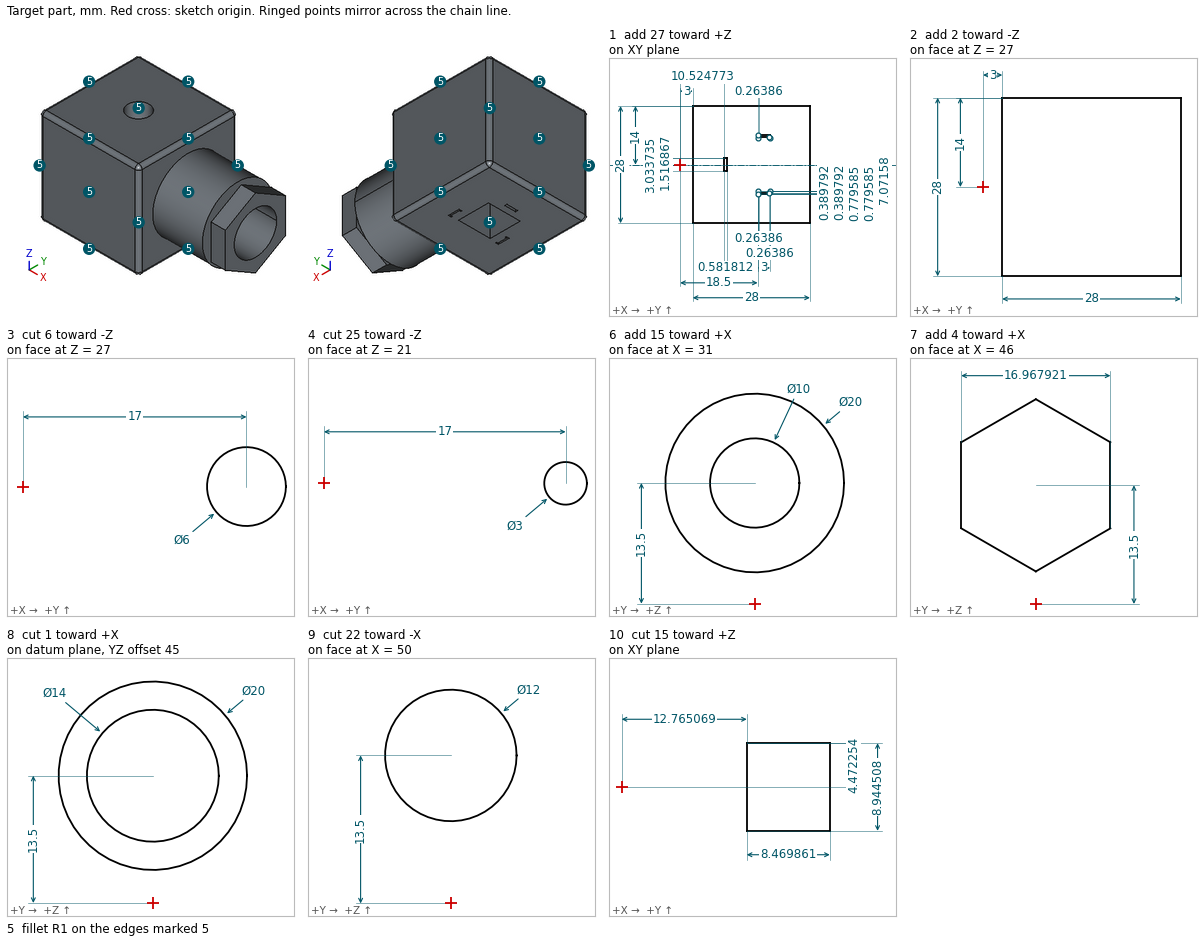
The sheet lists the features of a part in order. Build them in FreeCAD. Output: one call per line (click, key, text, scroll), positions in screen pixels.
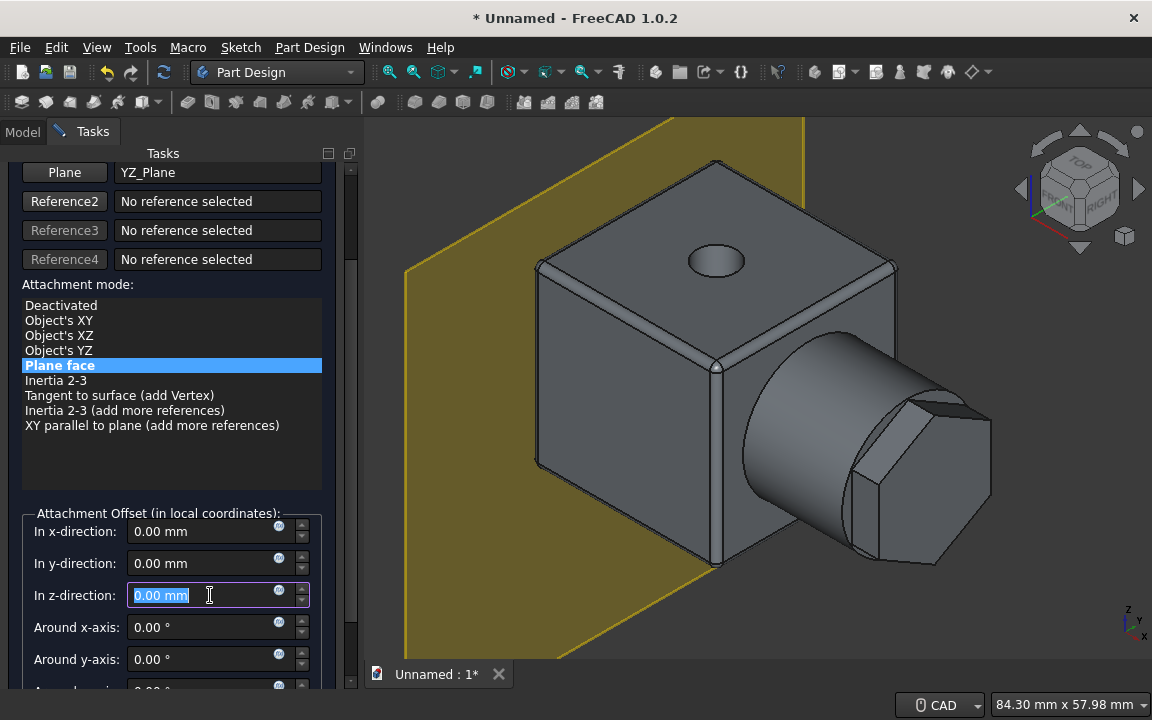
text(45)
key(Tab)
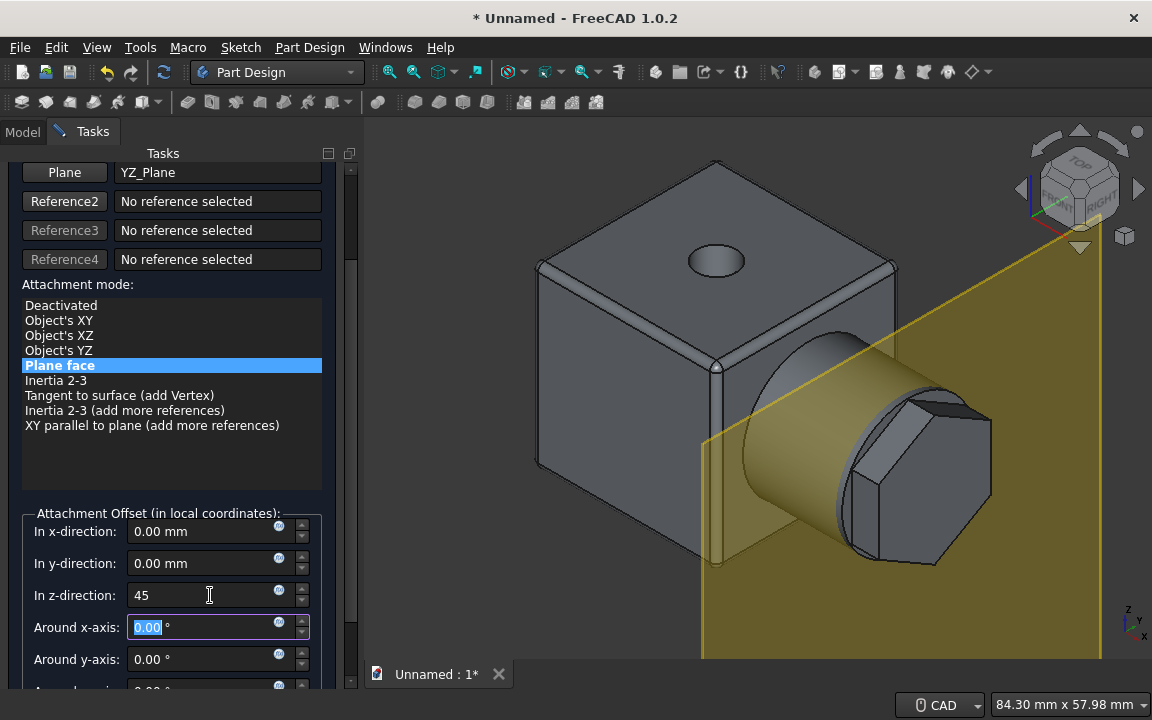
scroll(351, 426, up, 3)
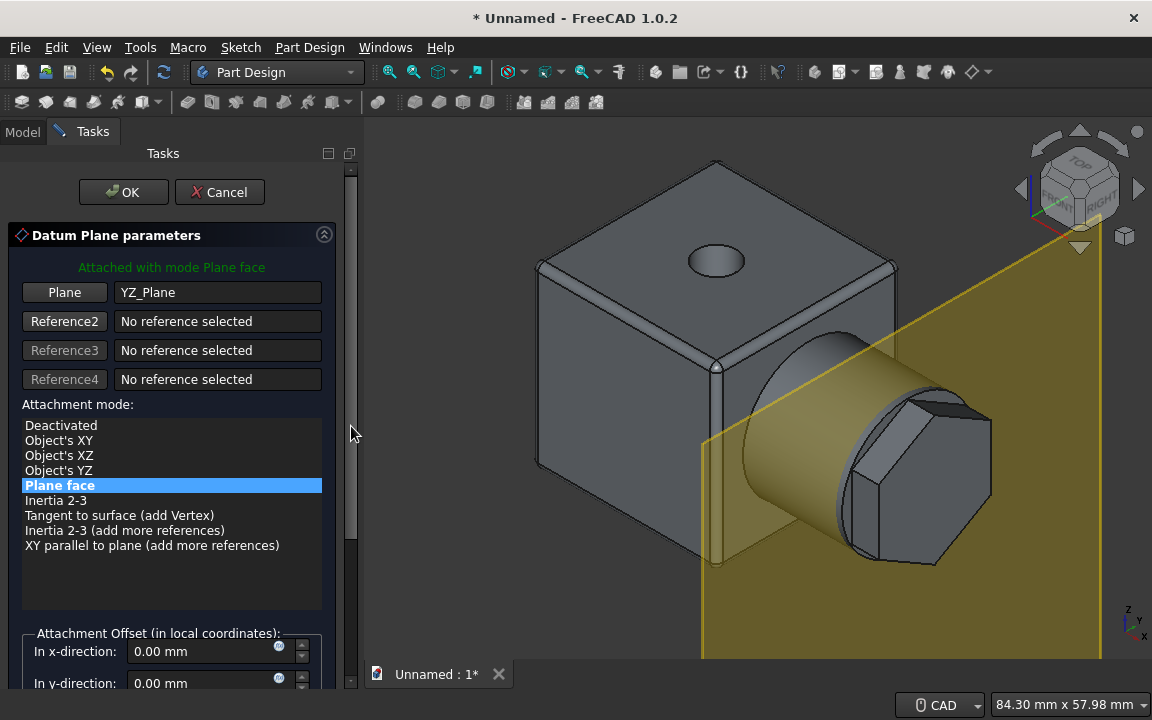
click(124, 192)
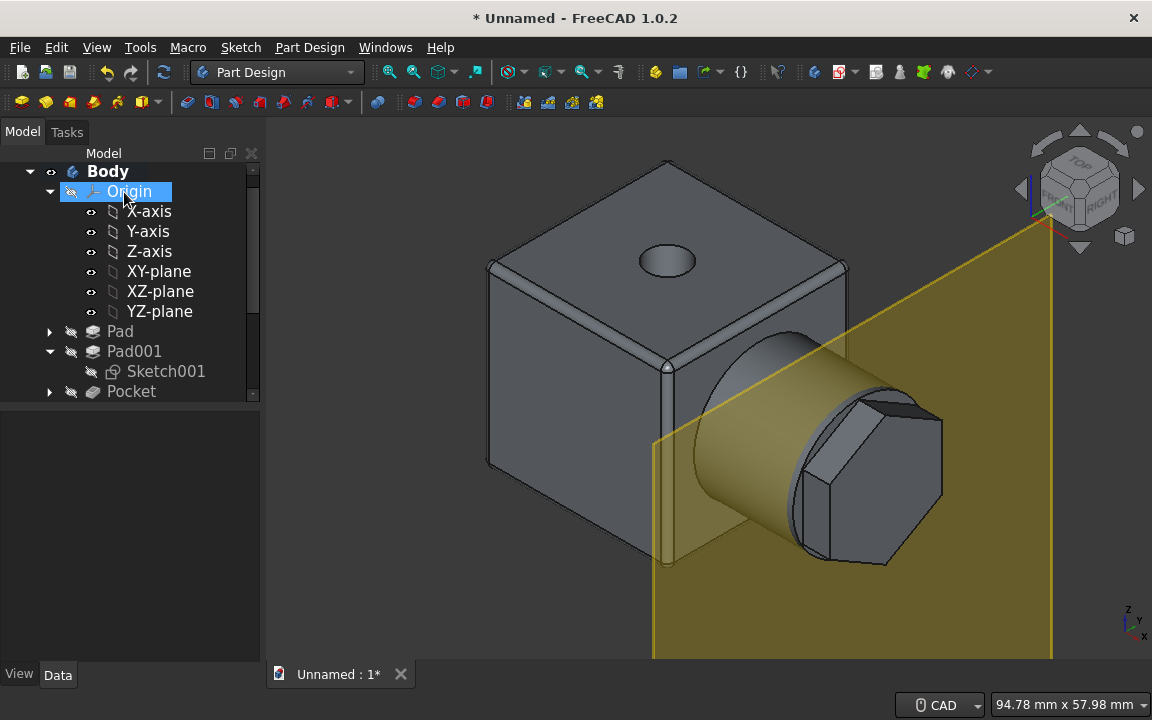
scroll(120, 287, down, 3)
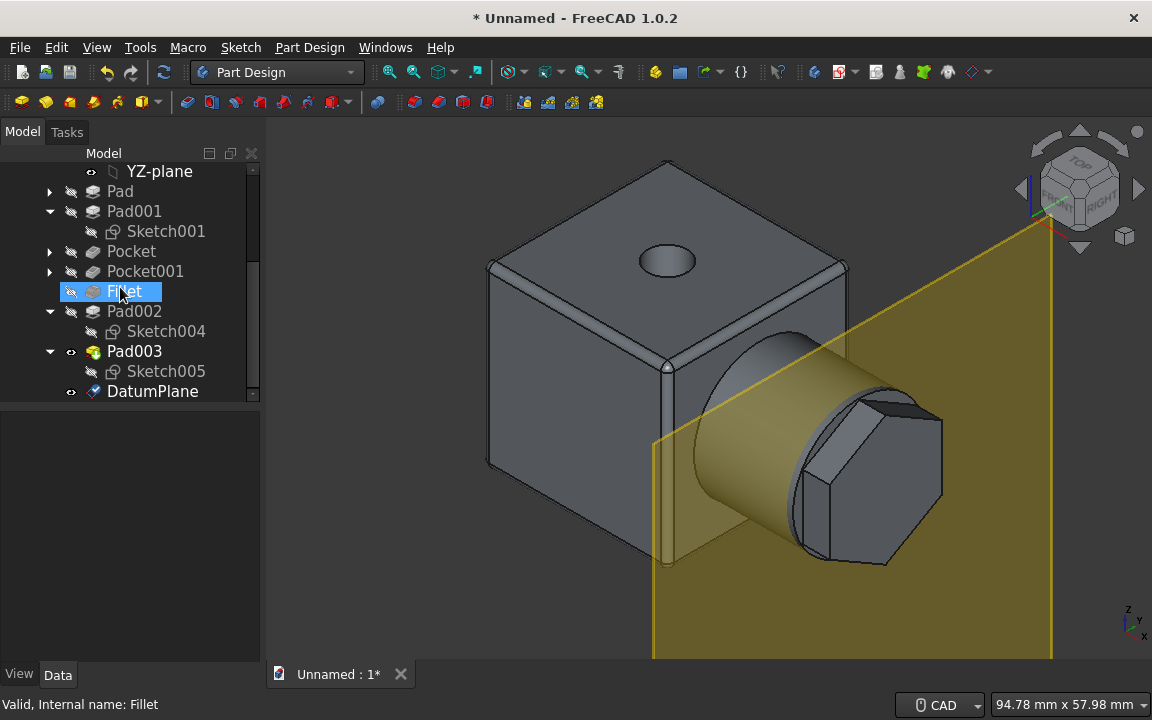
click(116, 392)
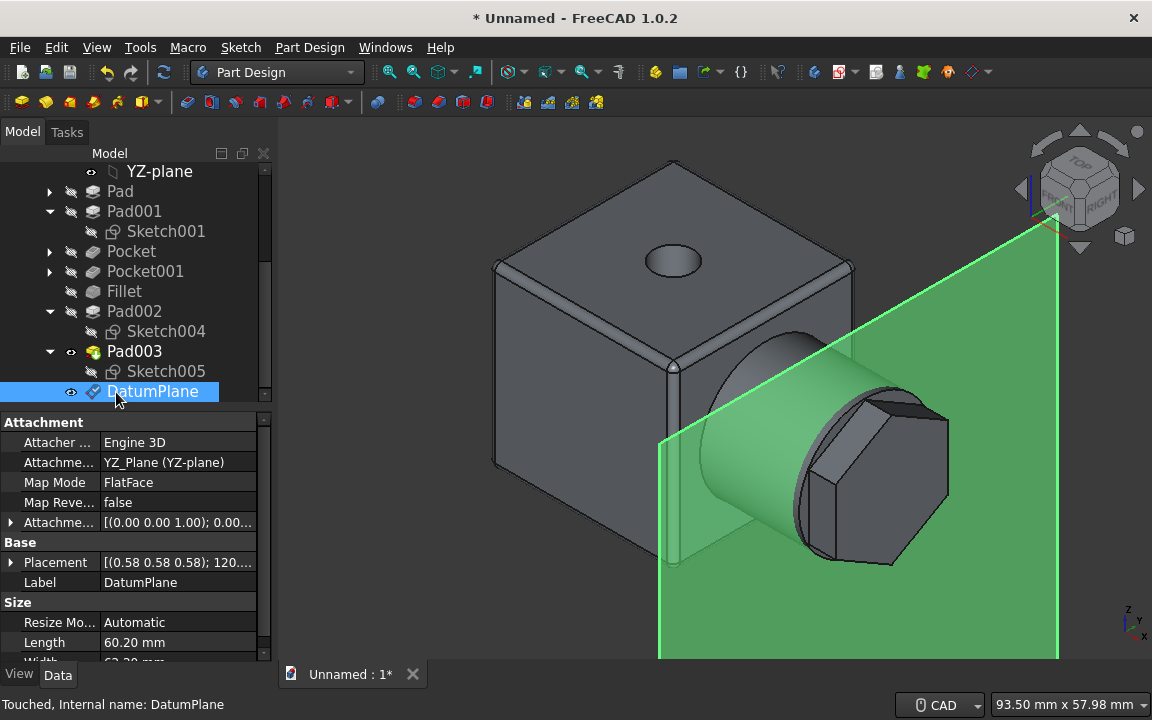
click(840, 72)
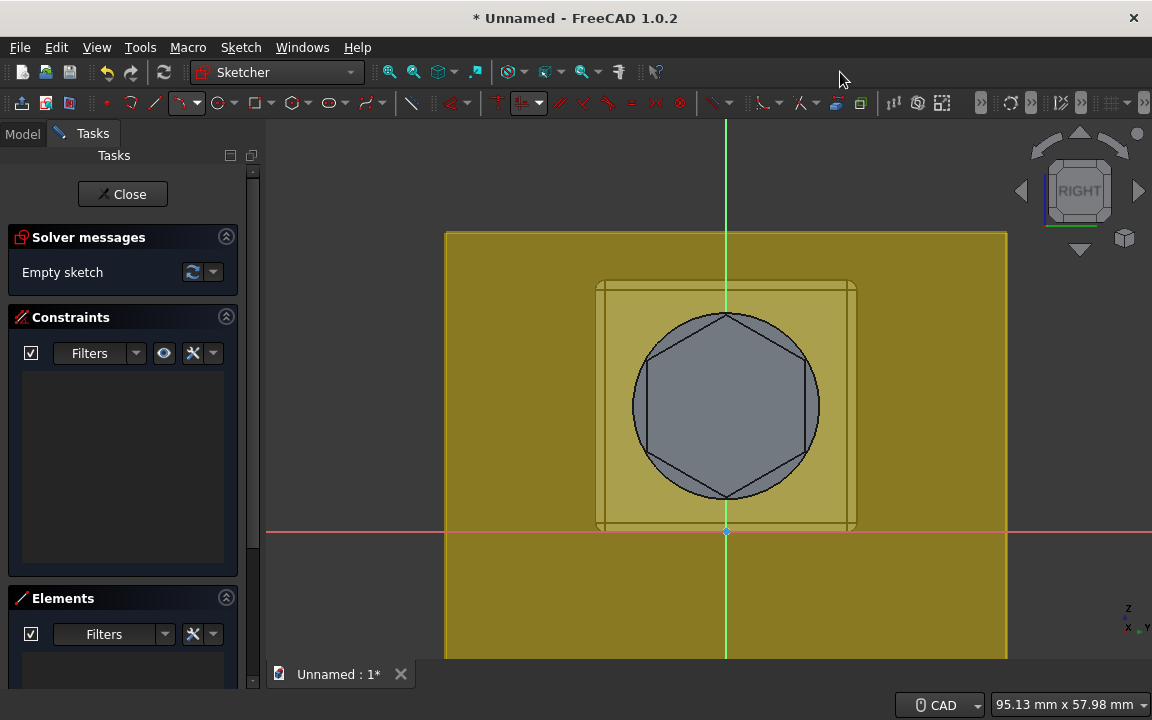
click(70, 104)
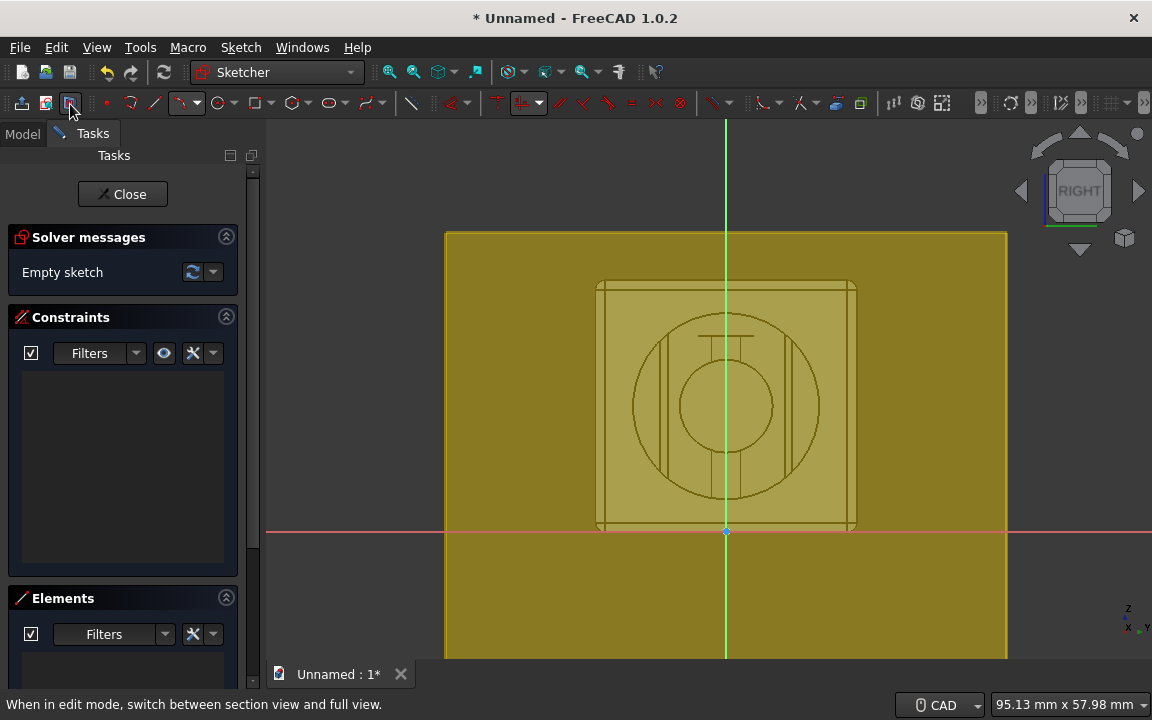
scroll(900, 491, up, 2)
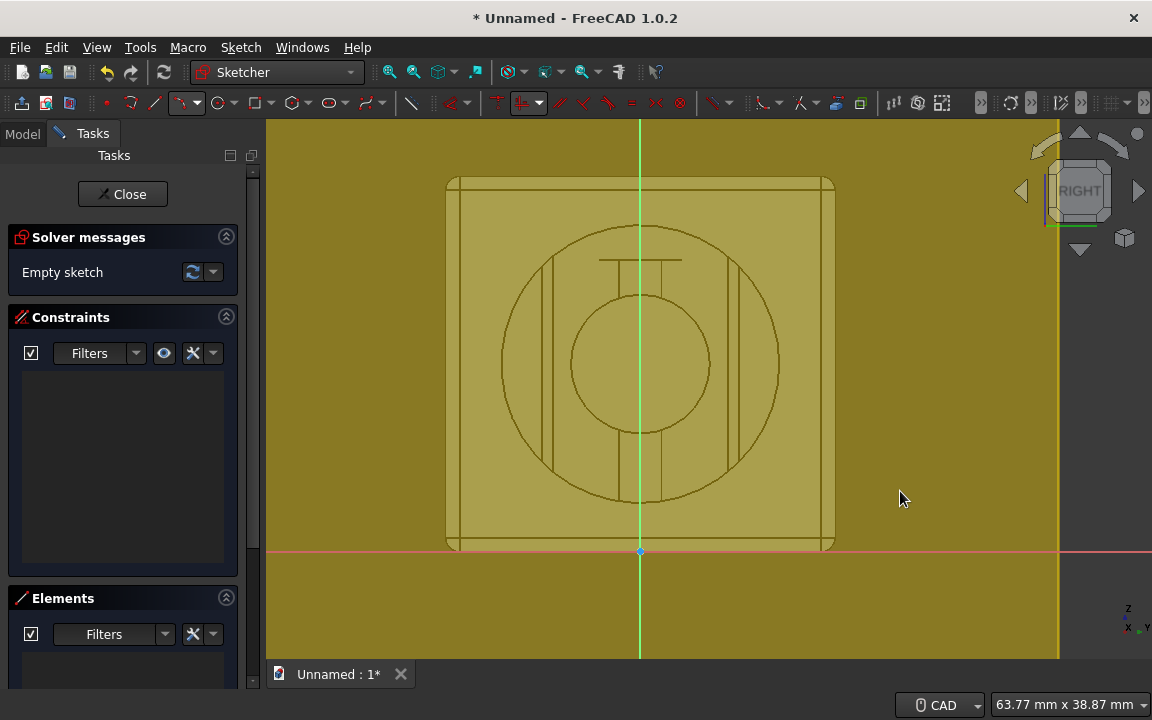
click(218, 104)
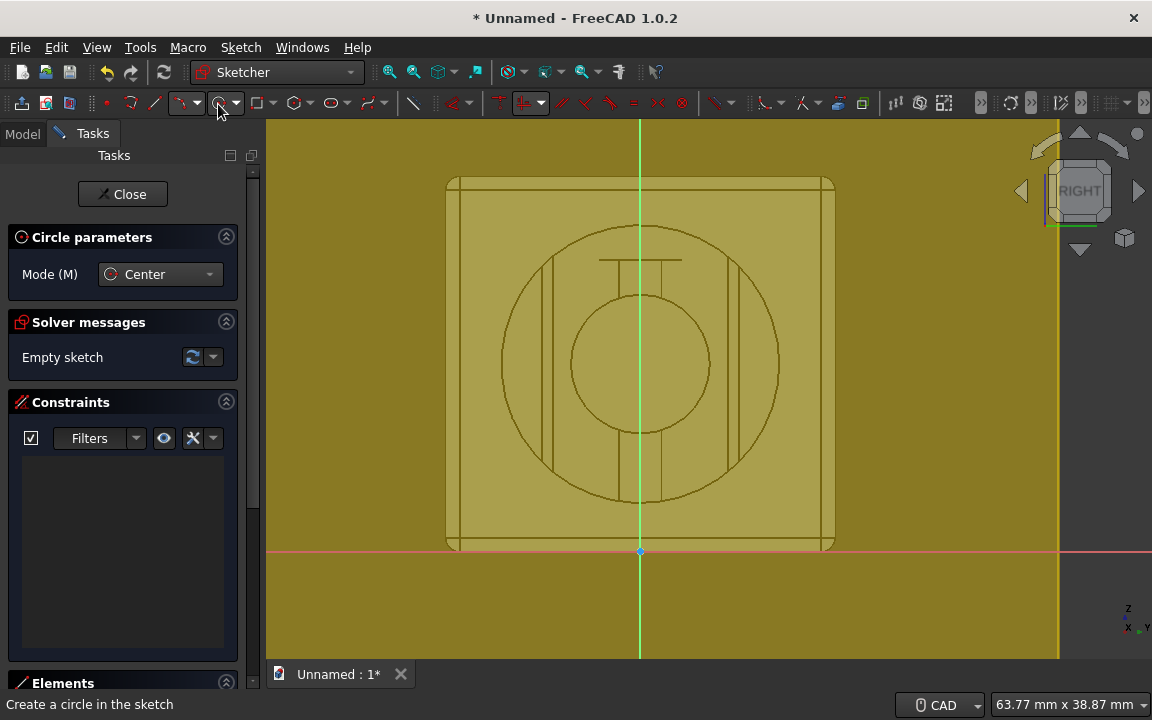
click(640, 364)
click(739, 266)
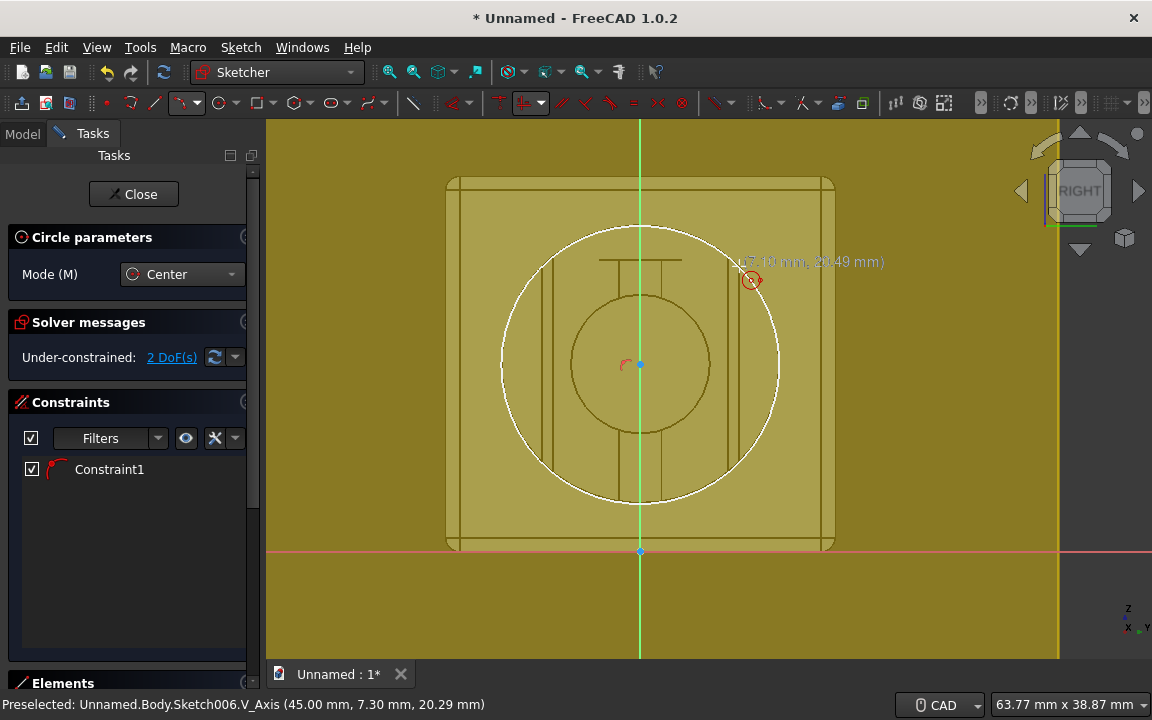
click(640, 365)
click(709, 295)
key(Escape)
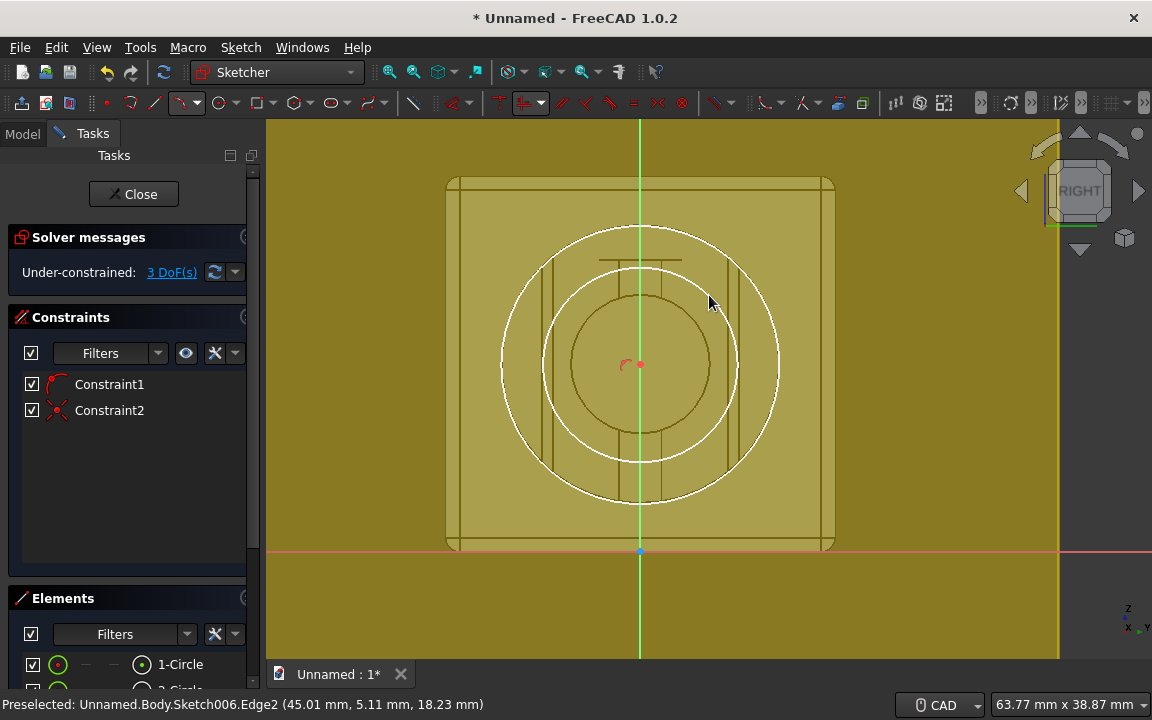
click(452, 104)